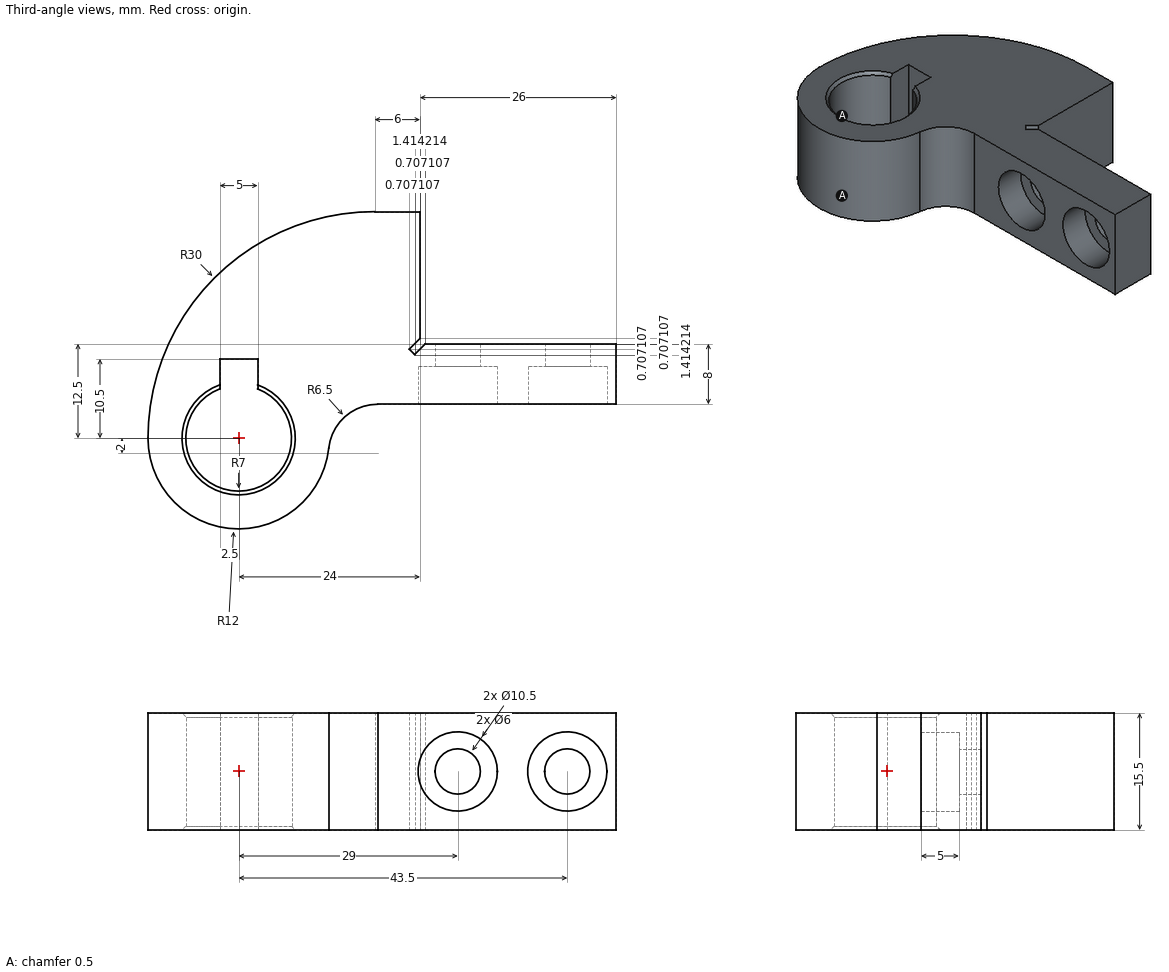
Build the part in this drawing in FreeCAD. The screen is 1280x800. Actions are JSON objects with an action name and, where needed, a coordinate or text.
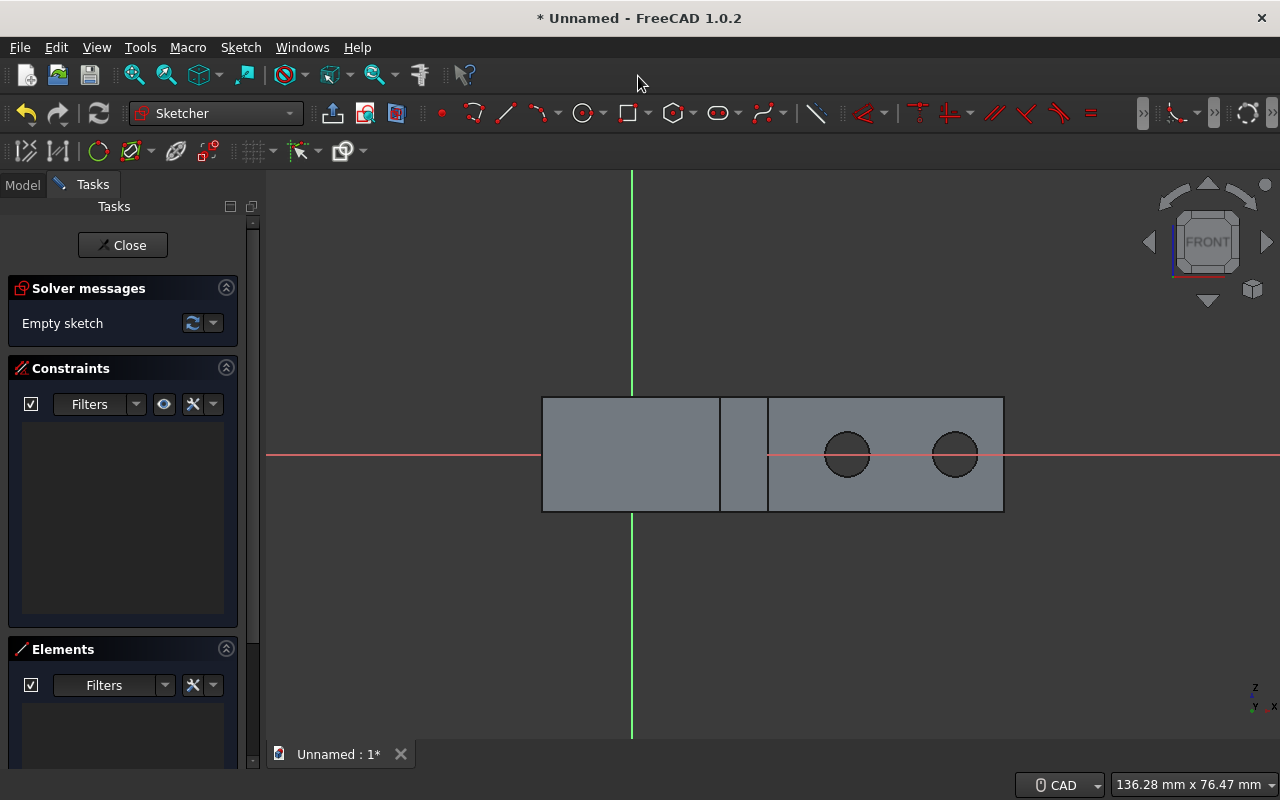
{"action": "scroll", "coordinate": [1034, 455], "scroll_direction": "up", "scroll_amount": 2}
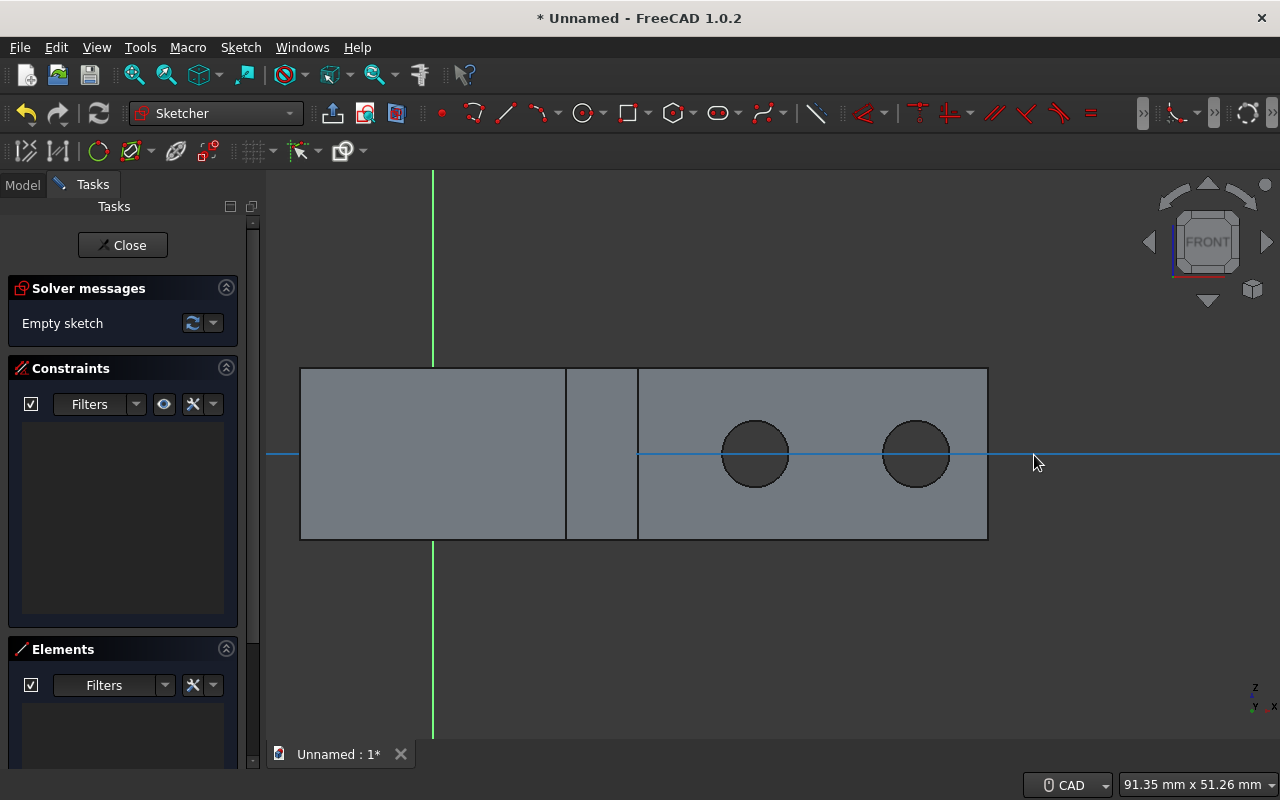
{"action": "left_click", "coordinate": [584, 114]}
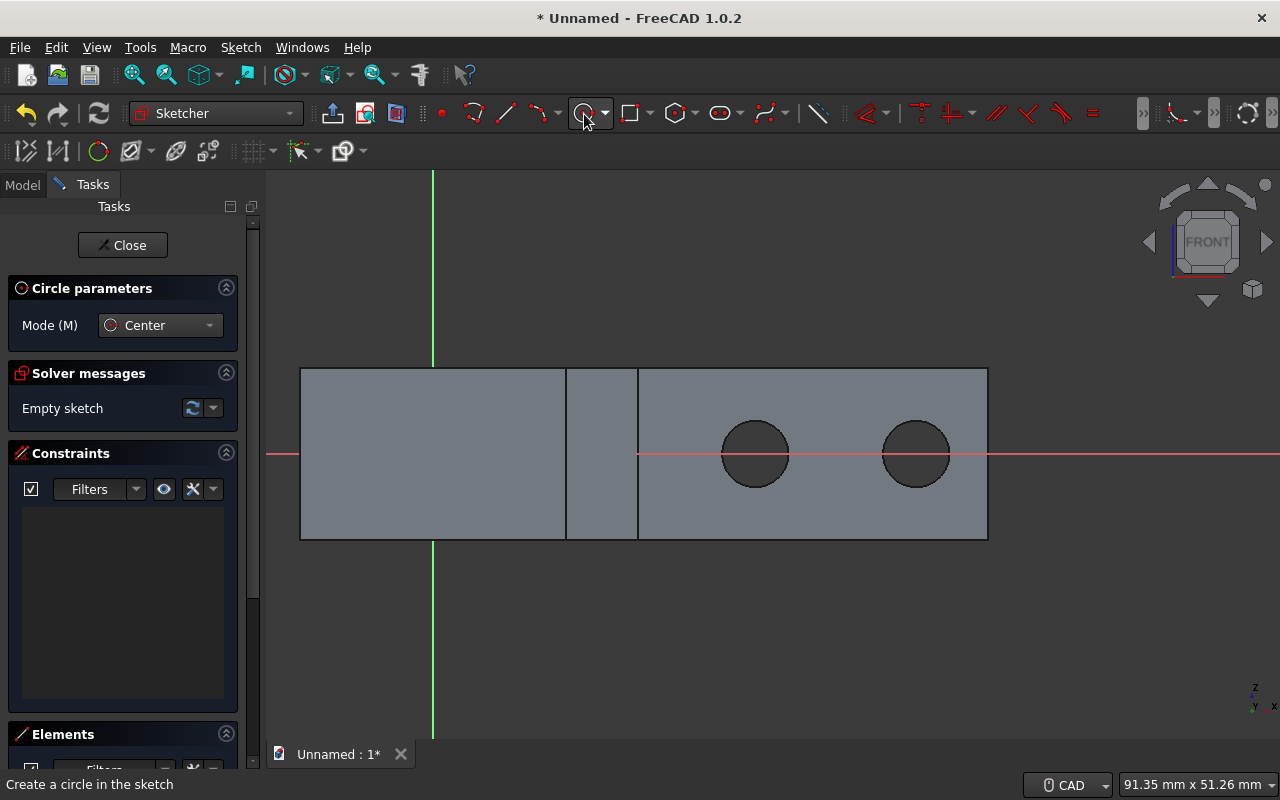
{"action": "left_click", "coordinate": [755, 454]}
{"action": "left_click", "coordinate": [796, 413]}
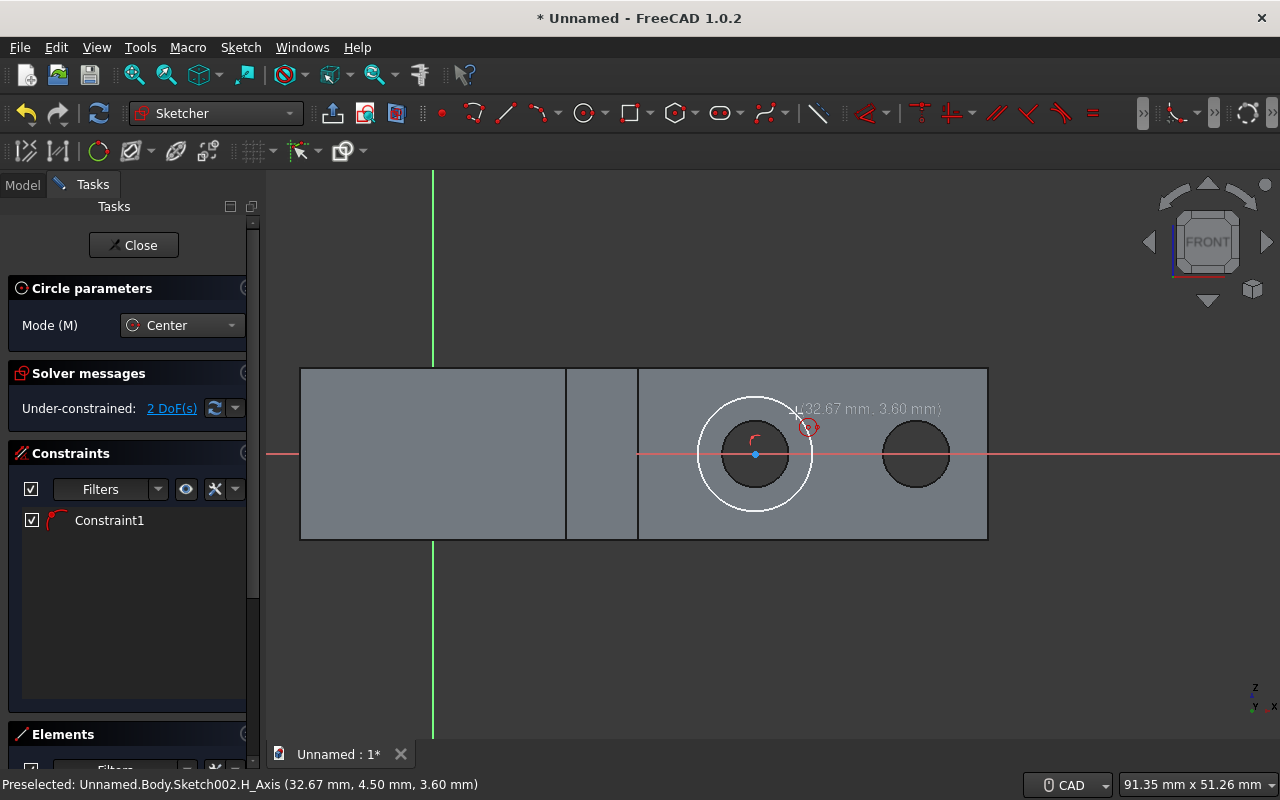
{"action": "left_click", "coordinate": [916, 454]}
{"action": "left_click", "coordinate": [957, 413]}
{"action": "key", "text": "Escape"}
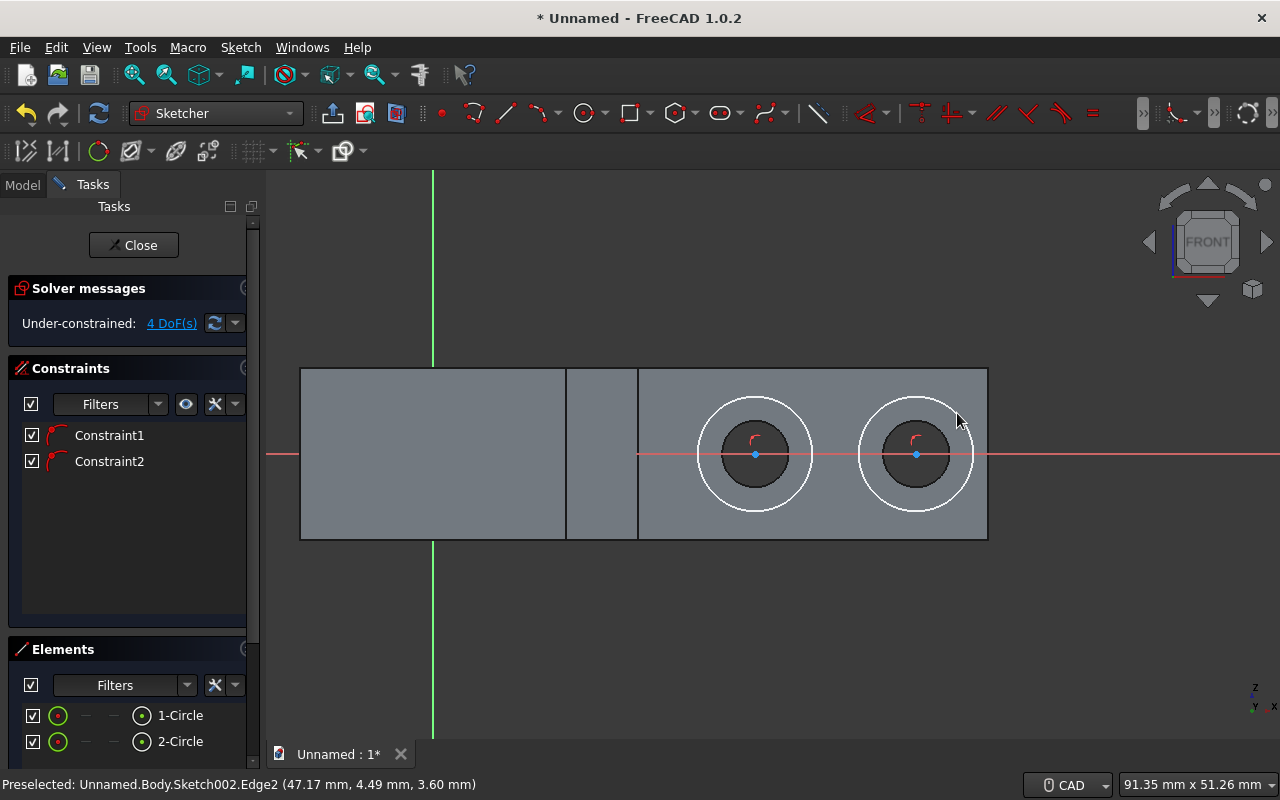
{"action": "left_click", "coordinate": [795, 413]}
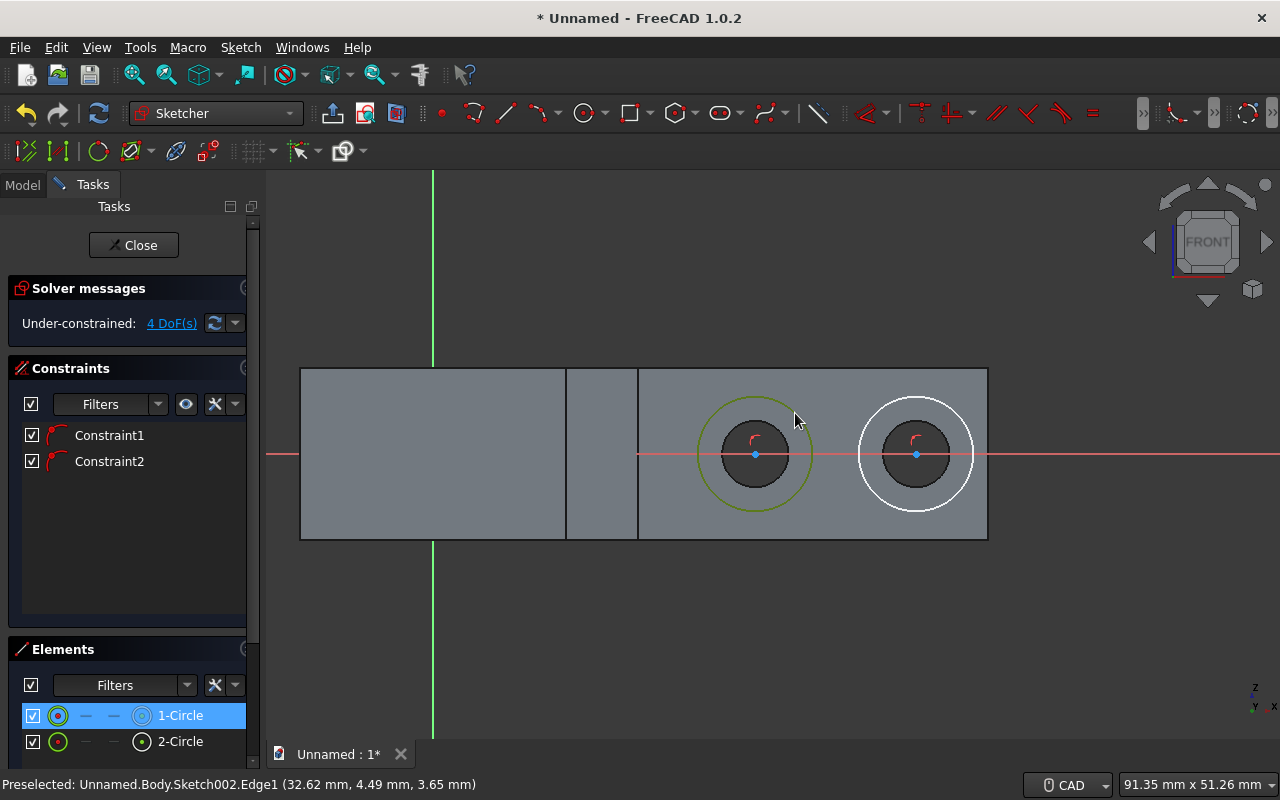
{"action": "left_click", "coordinate": [956, 413]}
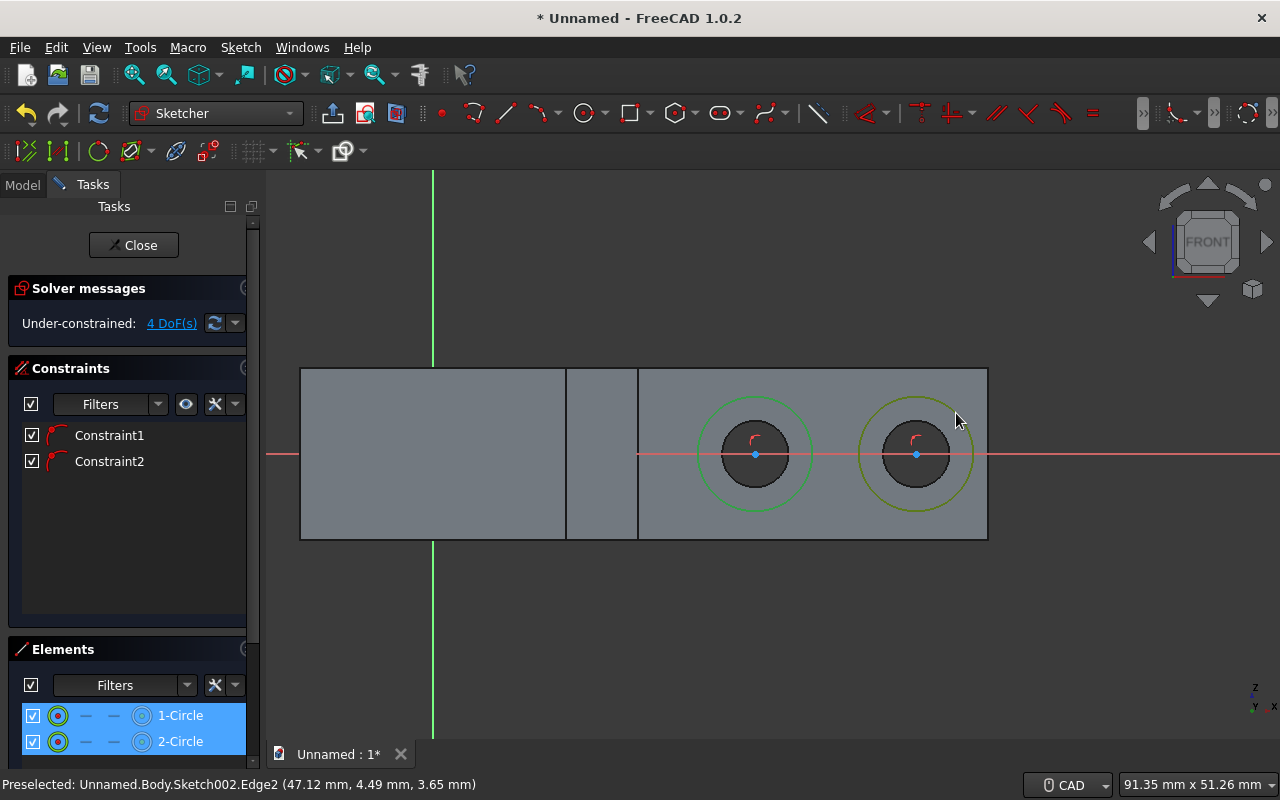
{"action": "left_click", "coordinate": [1094, 114]}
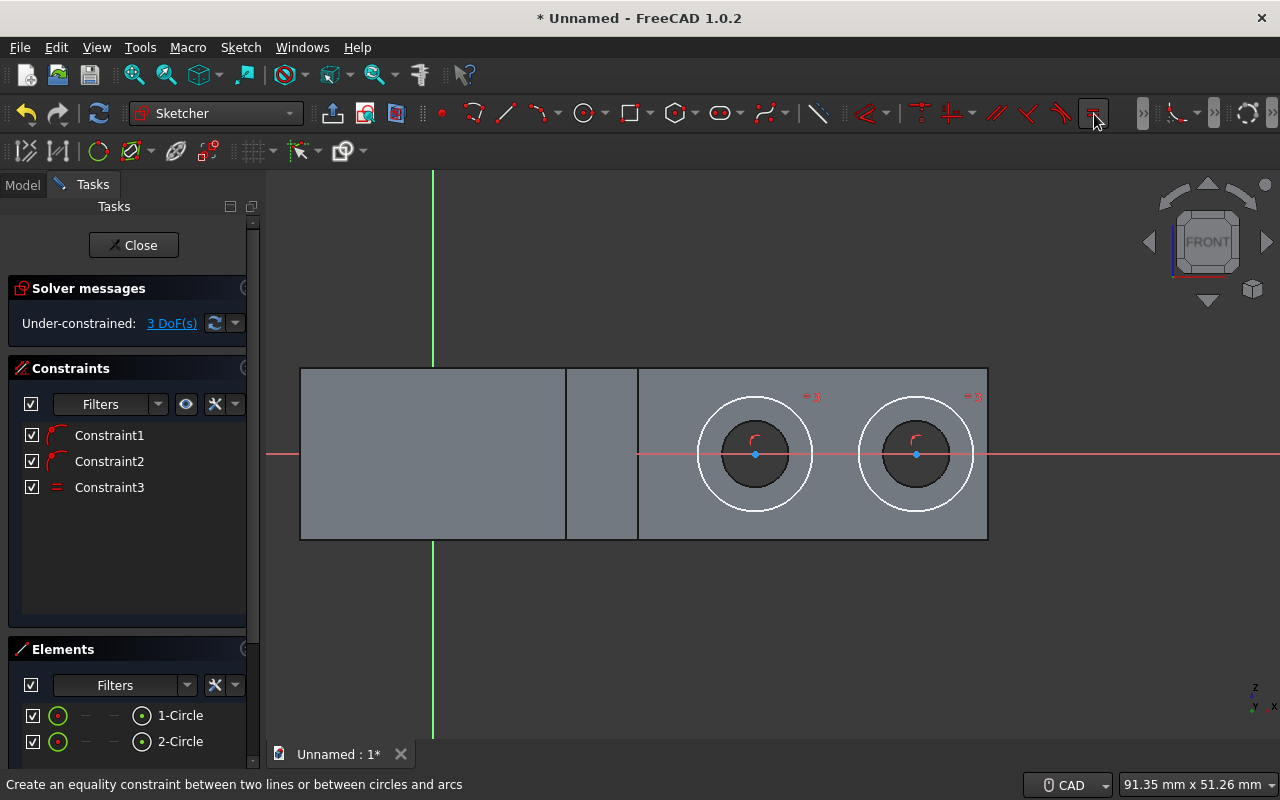
{"action": "key", "text": "d"}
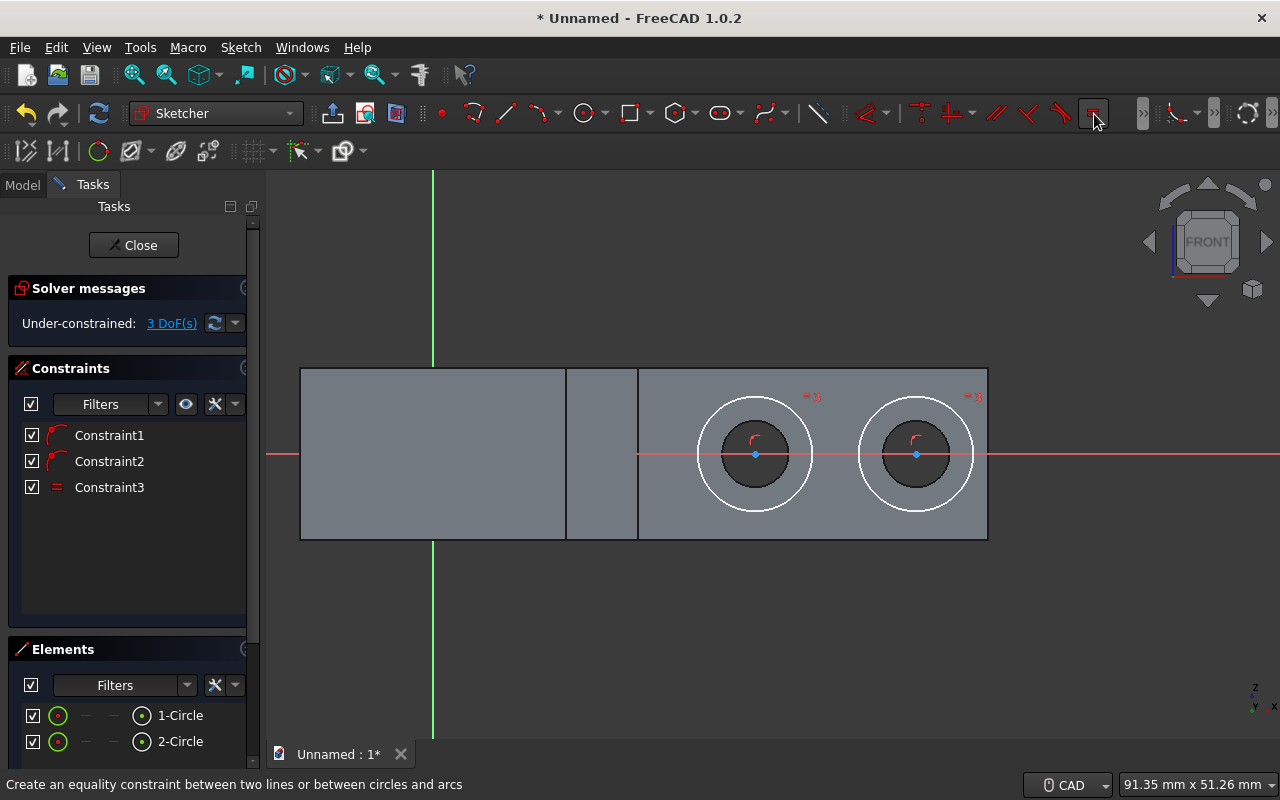
{"action": "left_click", "coordinate": [795, 413]}
{"action": "left_click", "coordinate": [817, 390]}